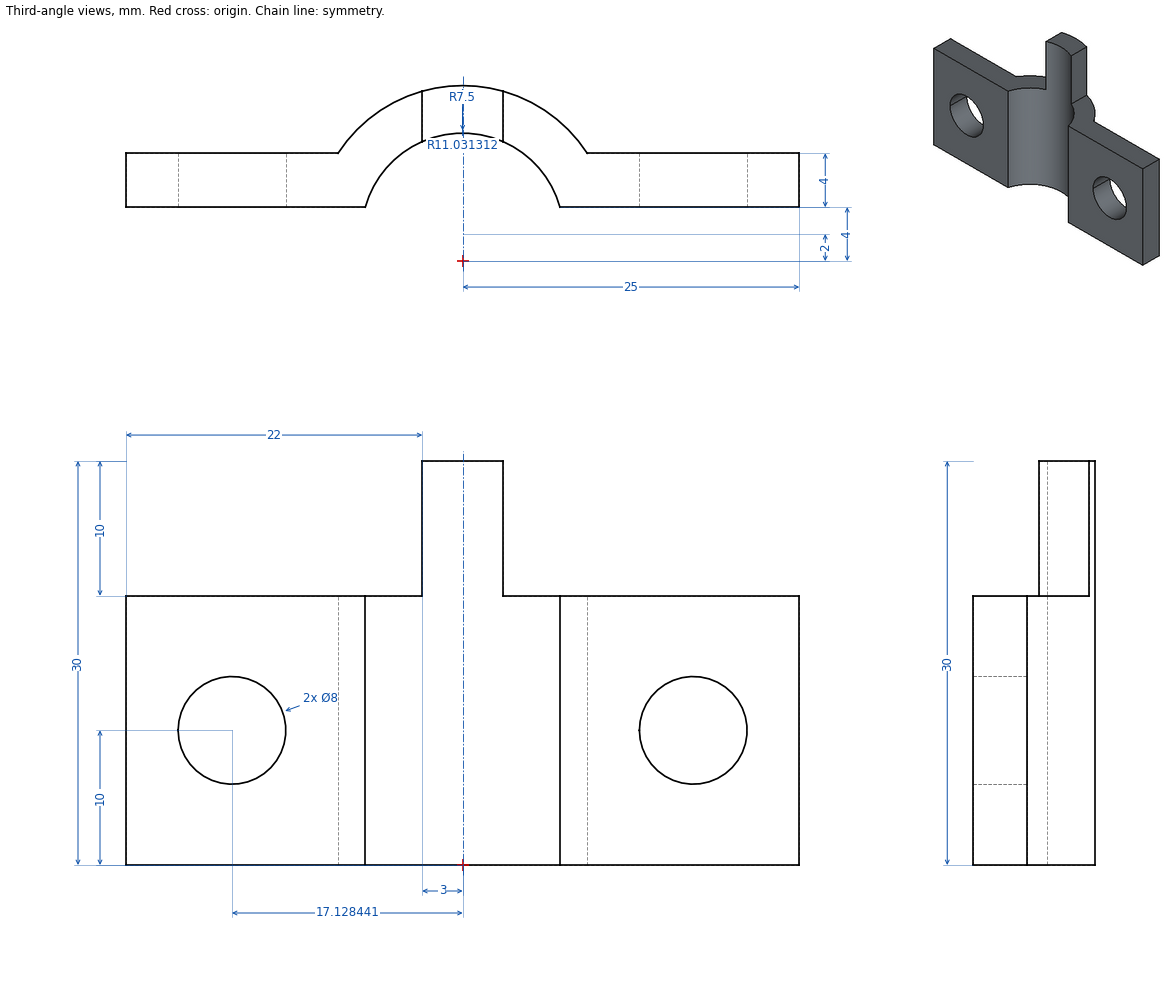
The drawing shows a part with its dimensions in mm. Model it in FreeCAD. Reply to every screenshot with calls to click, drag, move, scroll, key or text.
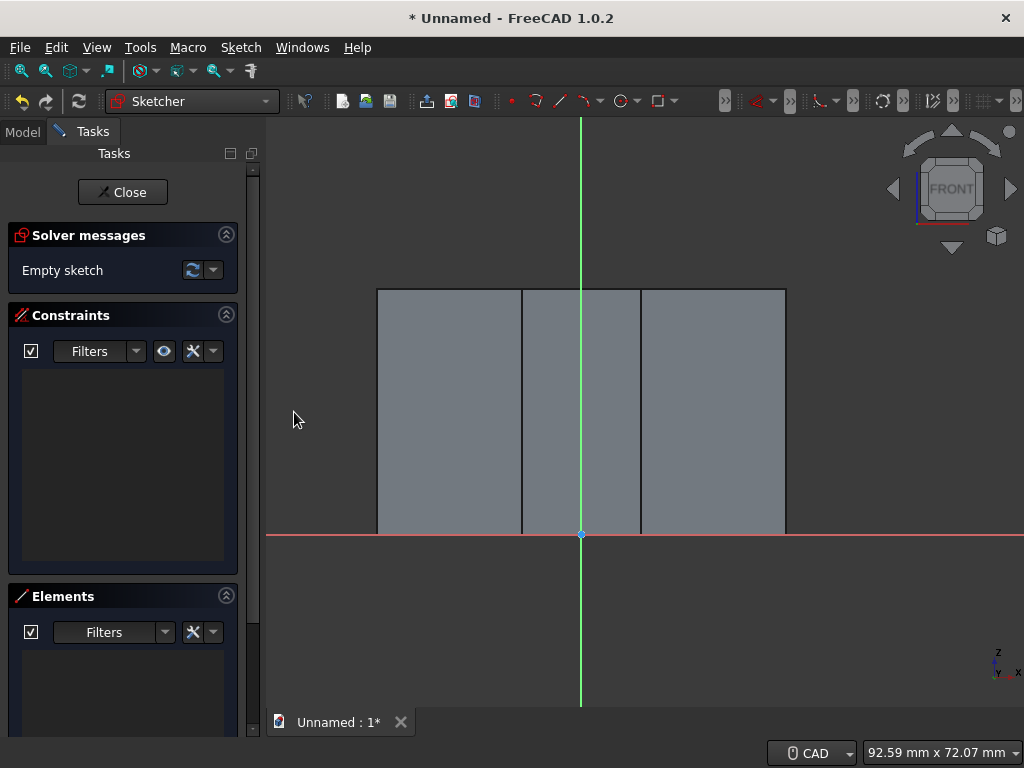
click(658, 102)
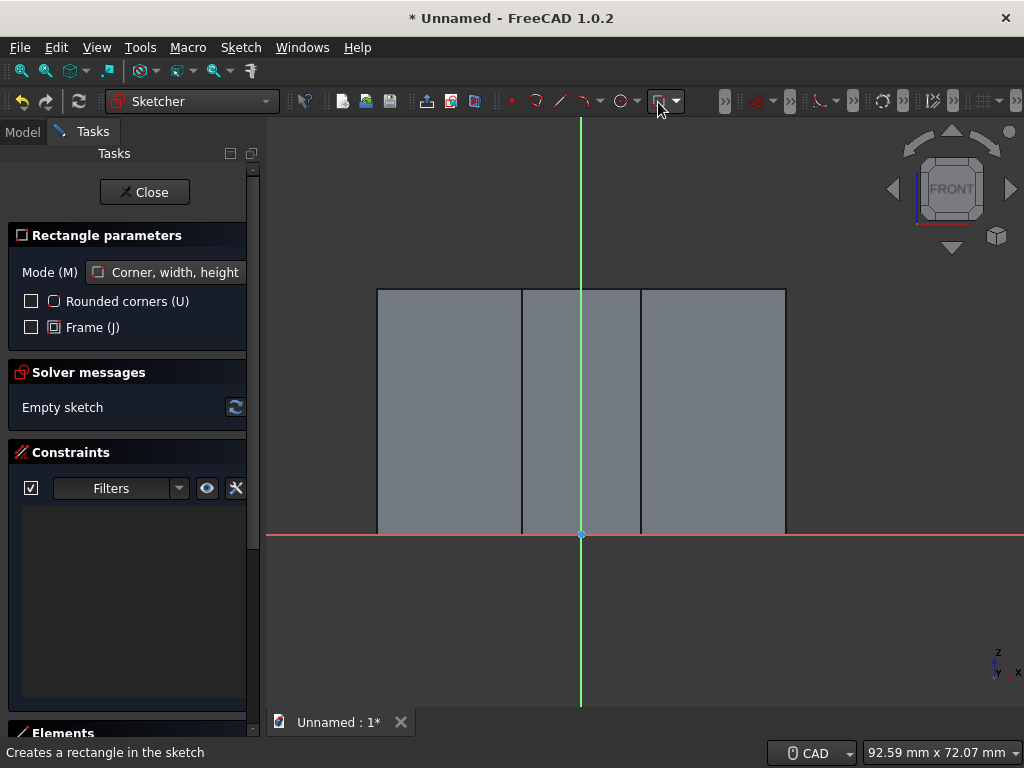
click(377, 289)
click(557, 371)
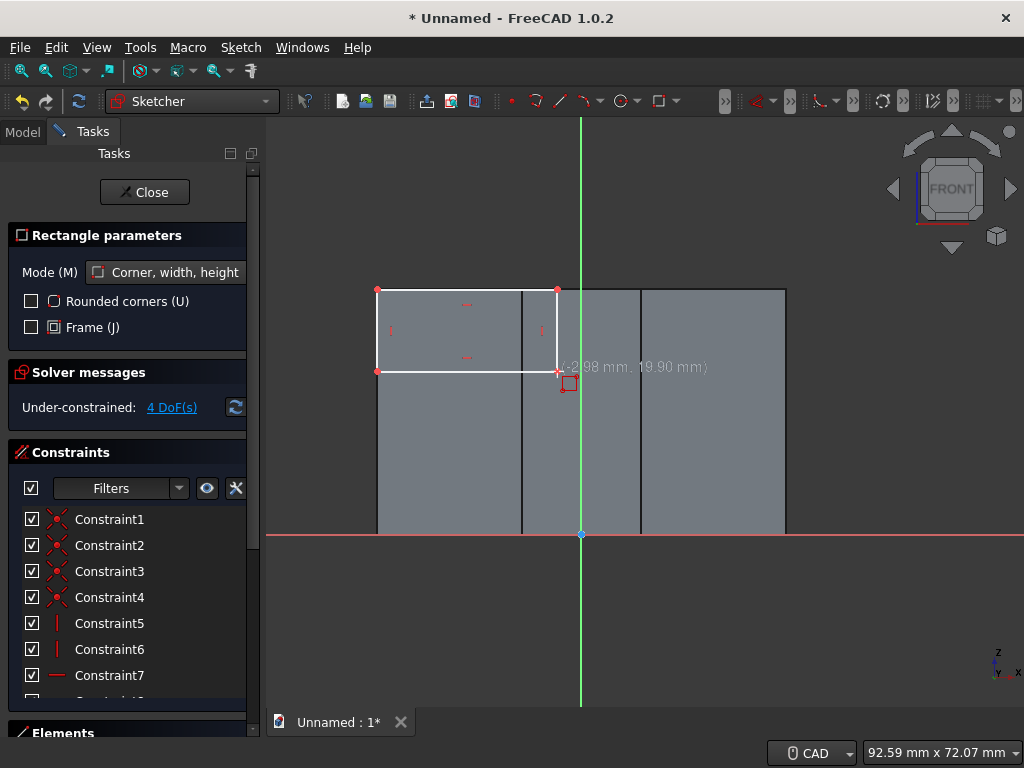
click(606, 289)
click(786, 371)
key(Escape)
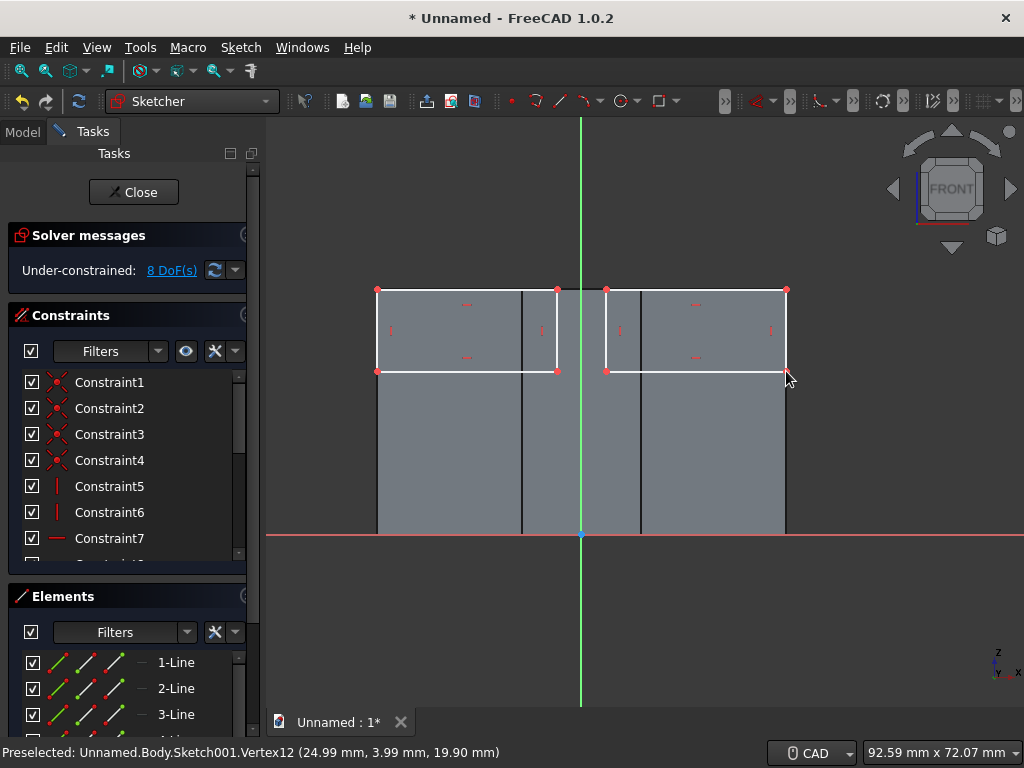
click(557, 290)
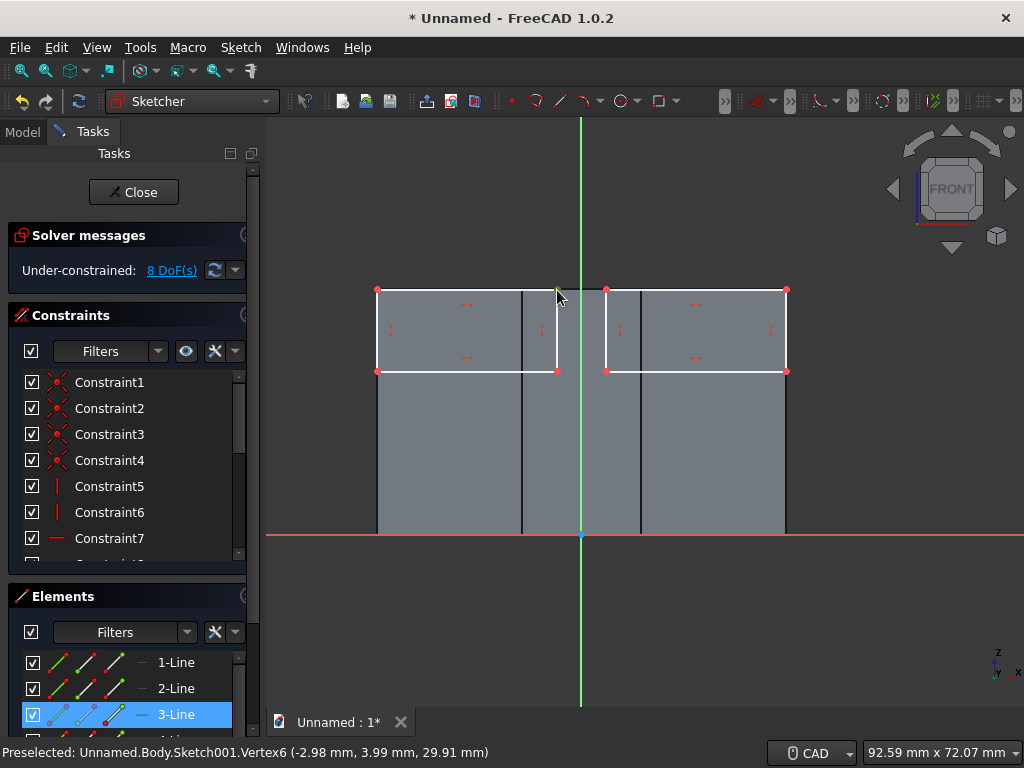
click(606, 290)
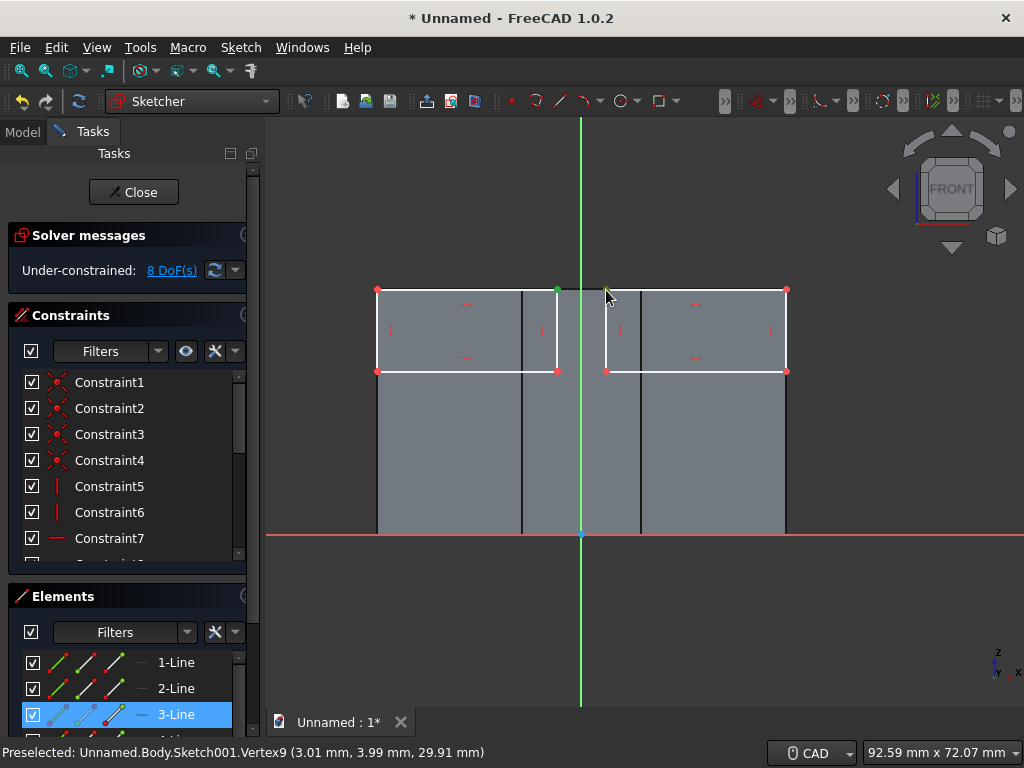
click(581, 641)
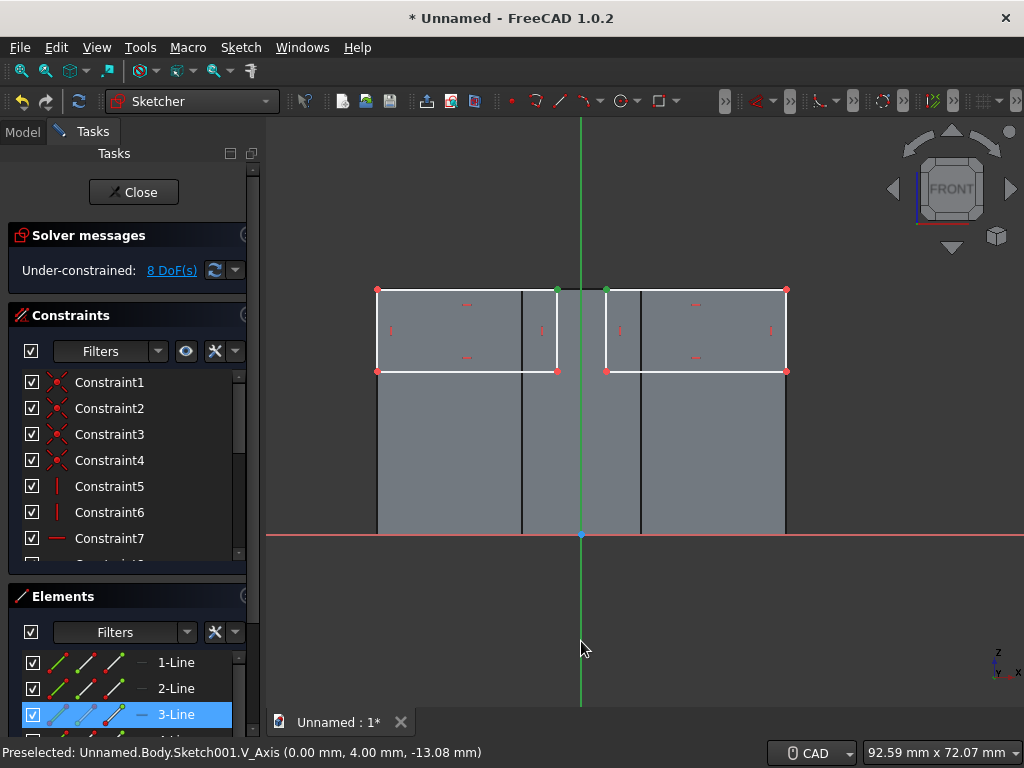
key(s)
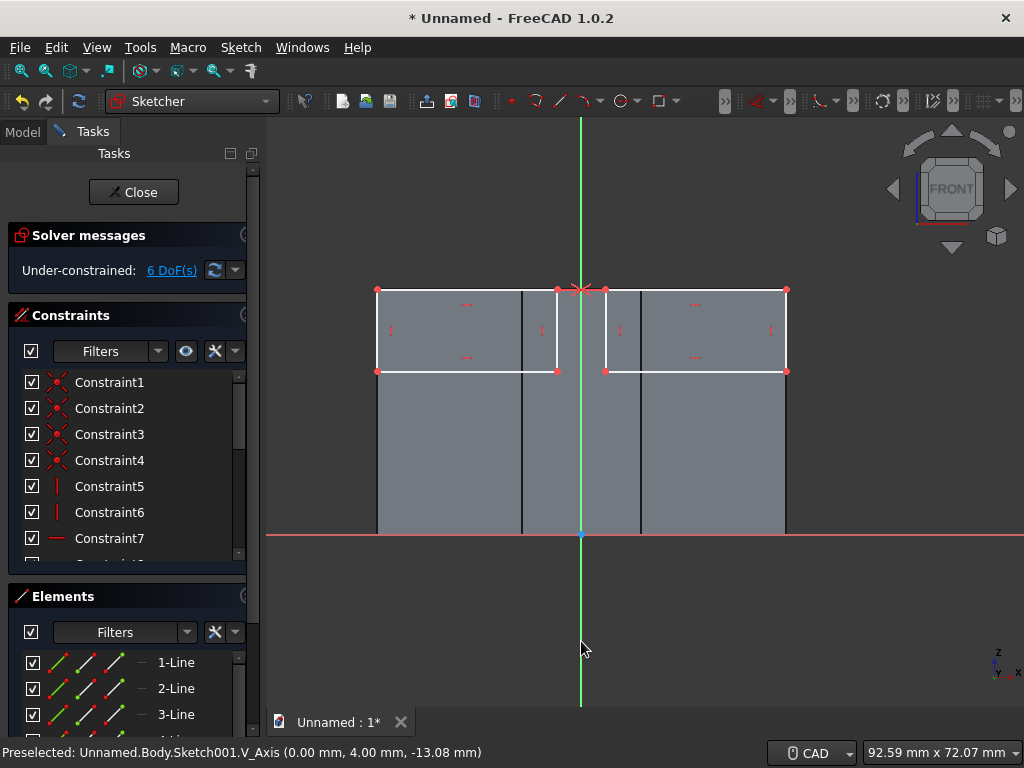
click(377, 372)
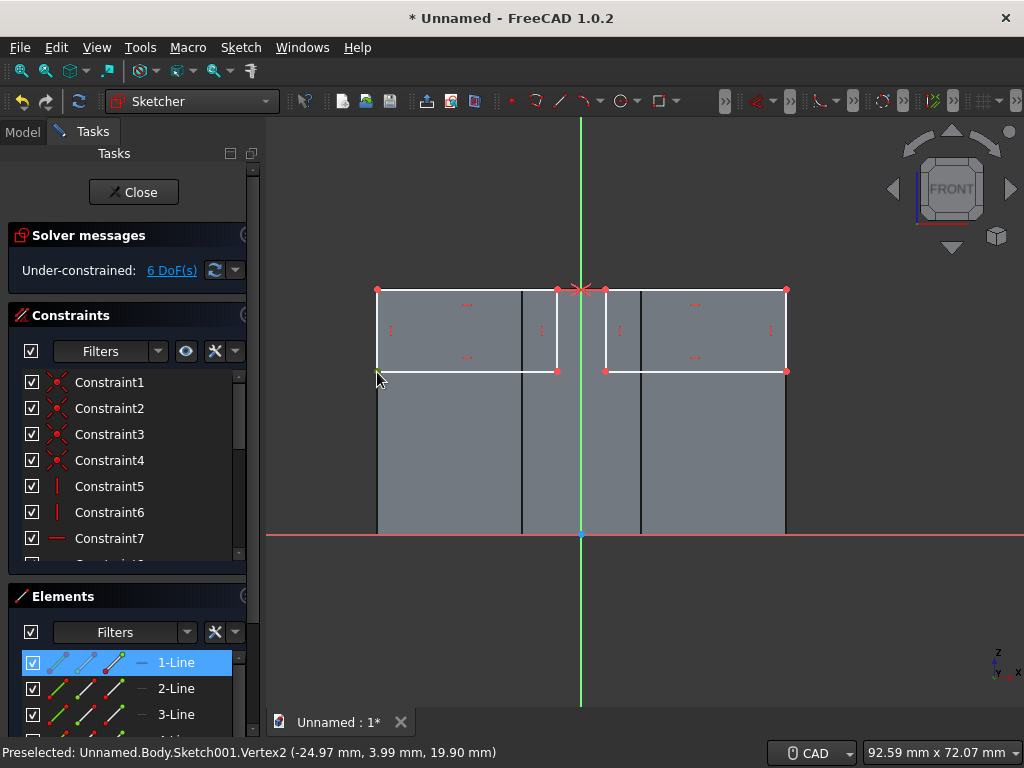
click(786, 372)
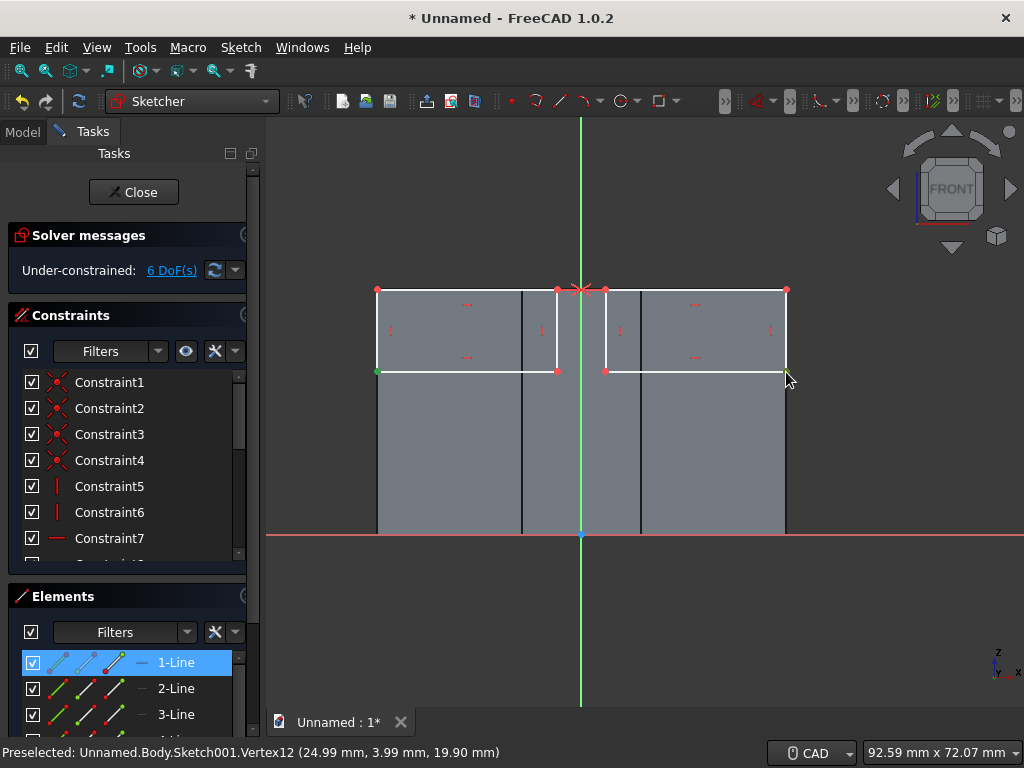
click(581, 641)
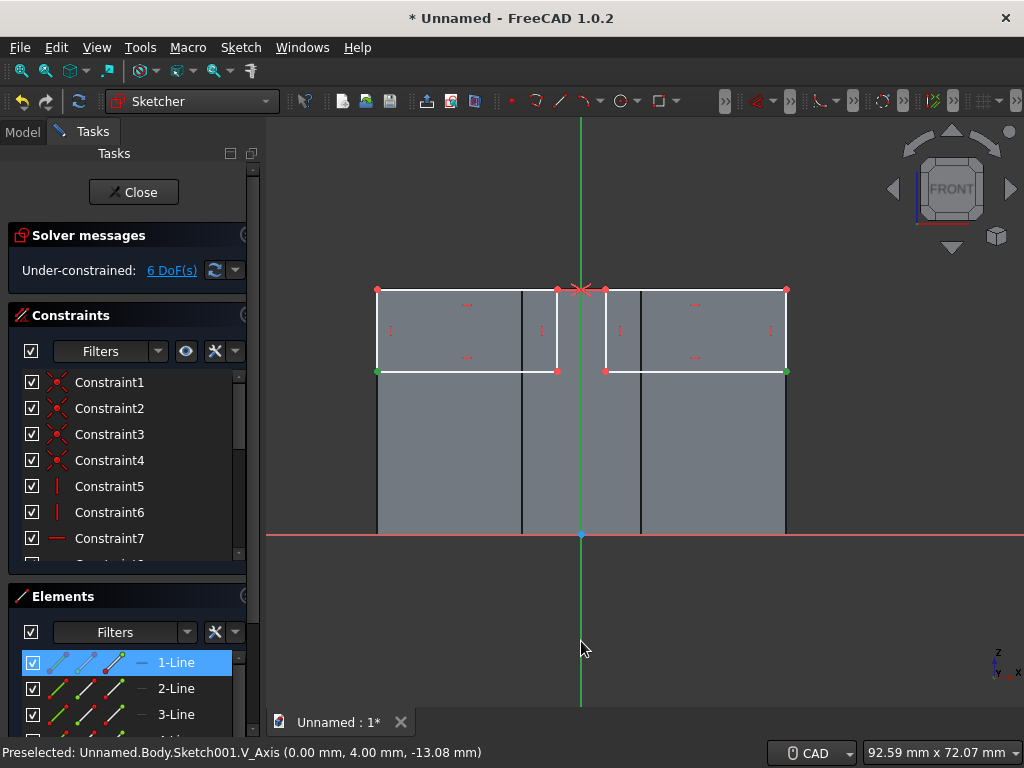
key(s)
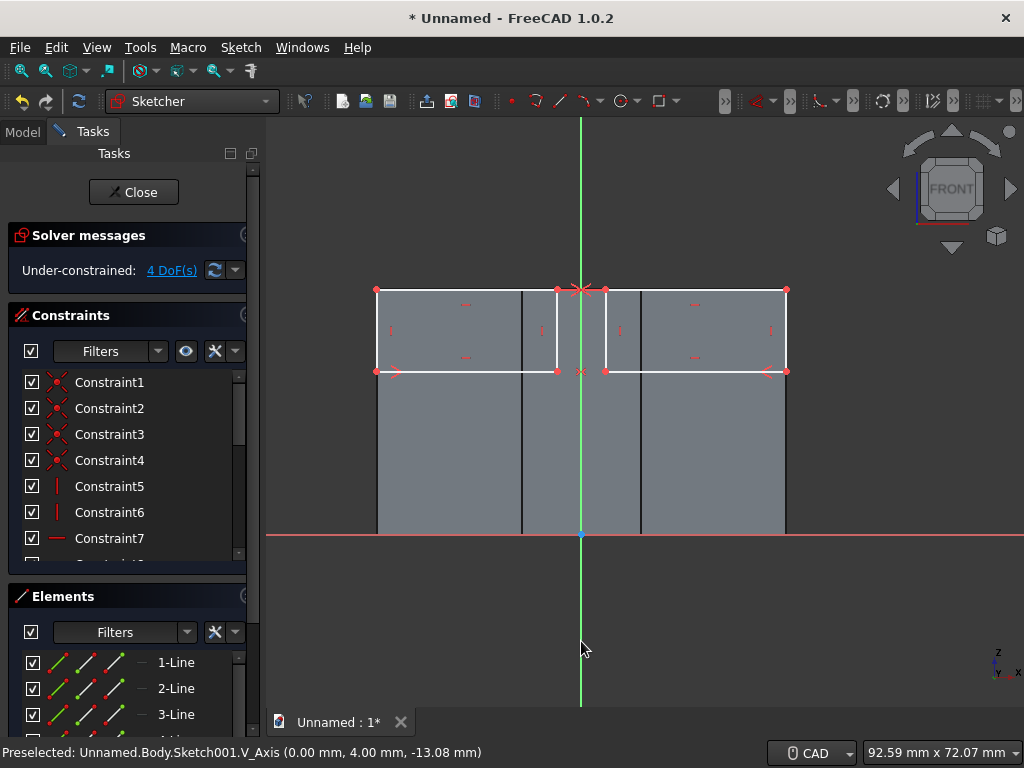
click(756, 102)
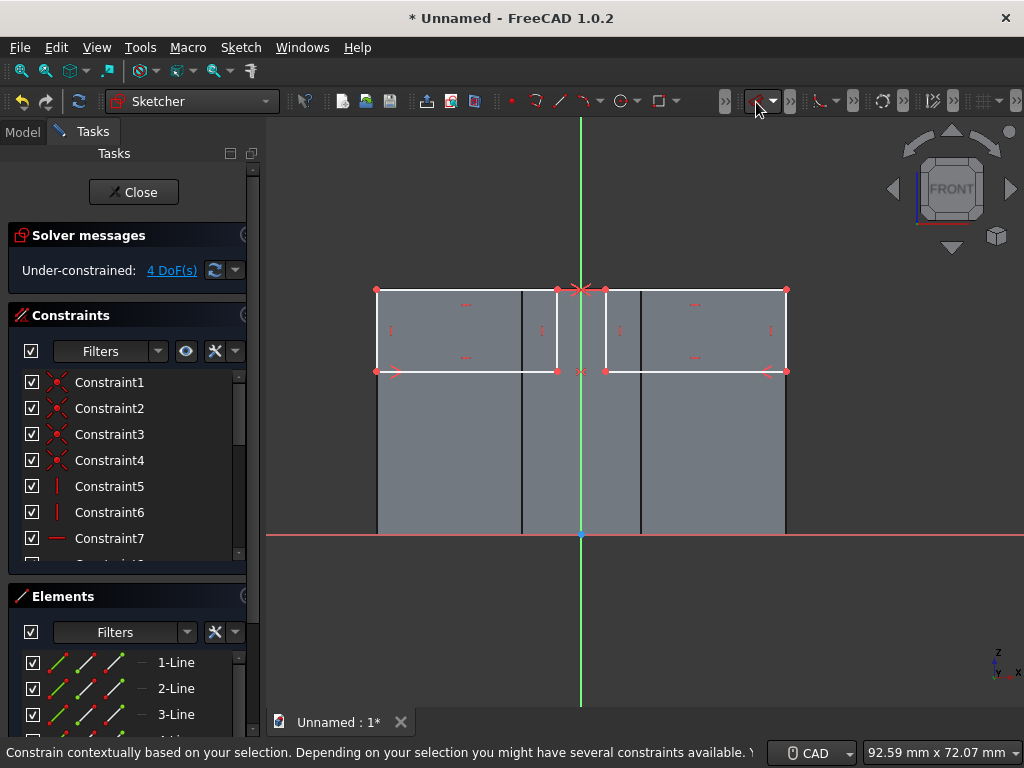
click(377, 315)
click(343, 331)